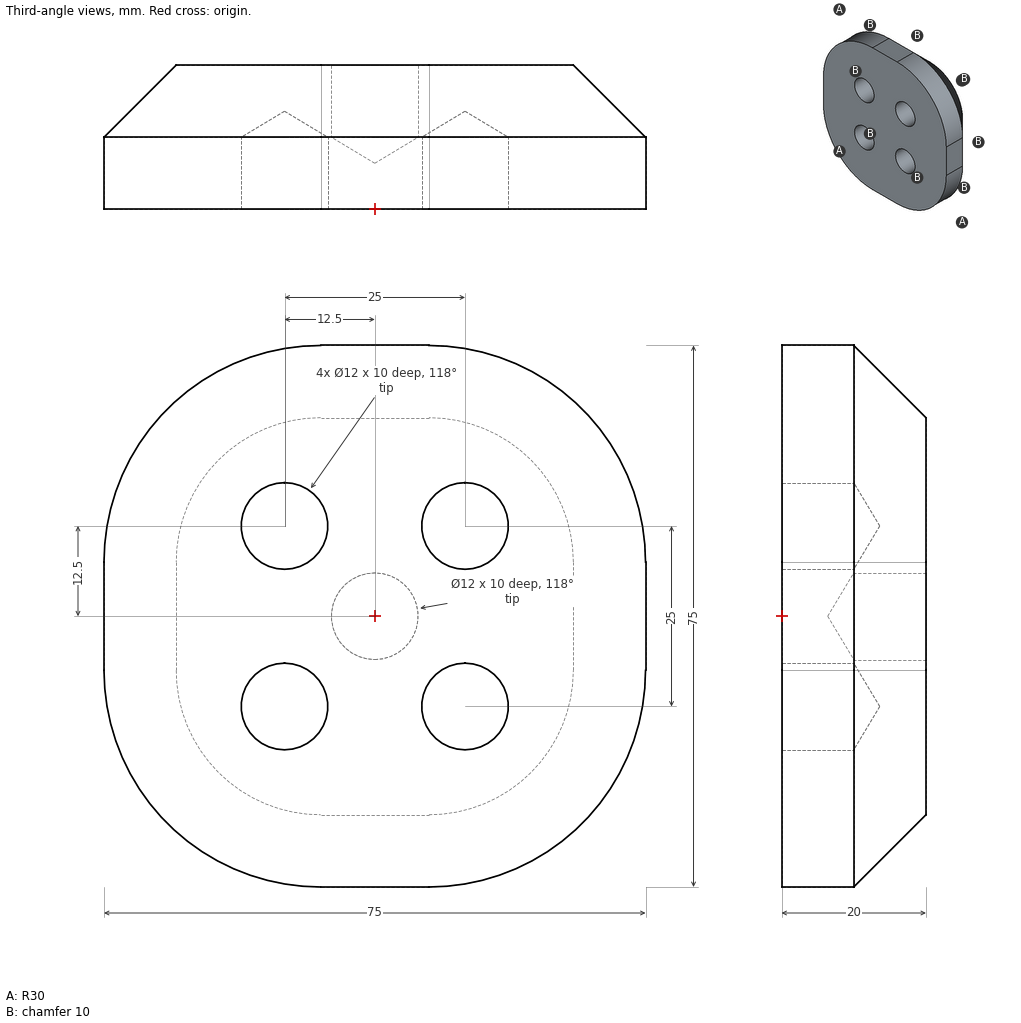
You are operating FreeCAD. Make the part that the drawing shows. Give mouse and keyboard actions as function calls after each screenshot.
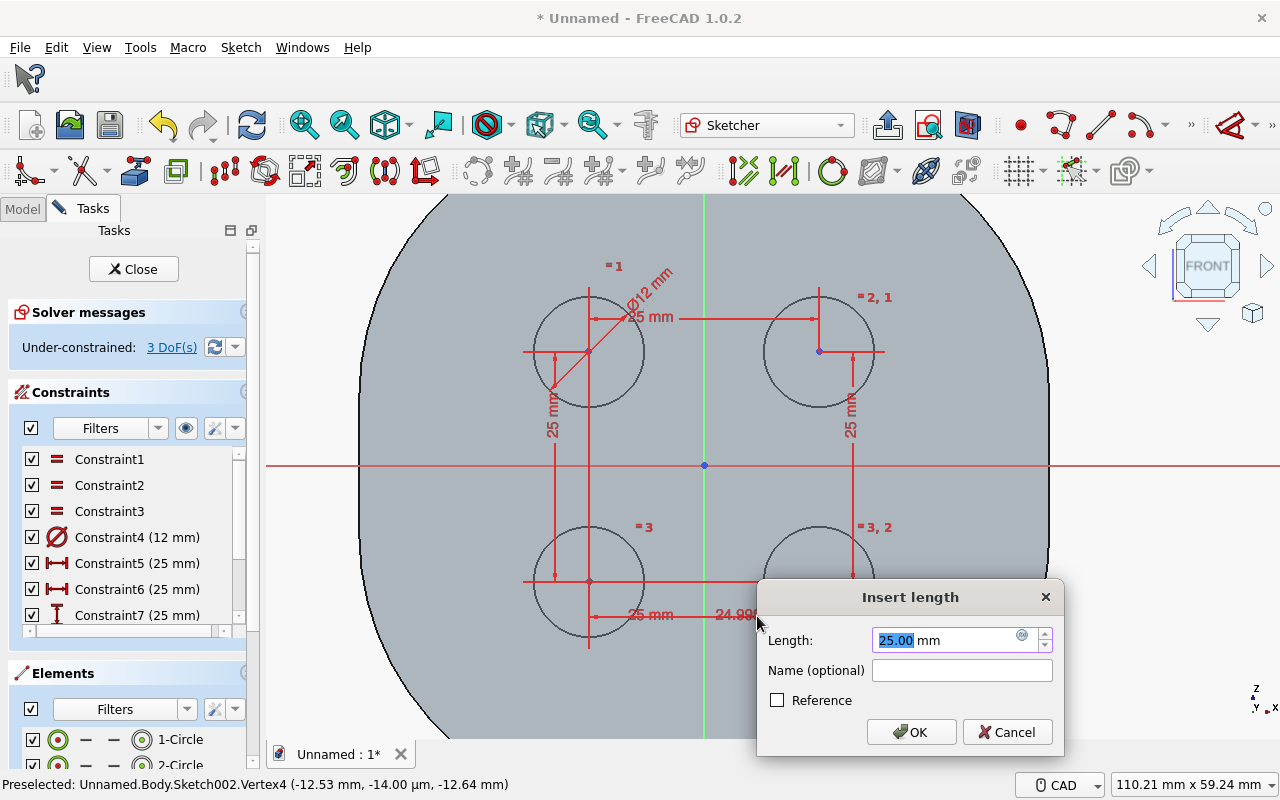
text(25)
key(Return)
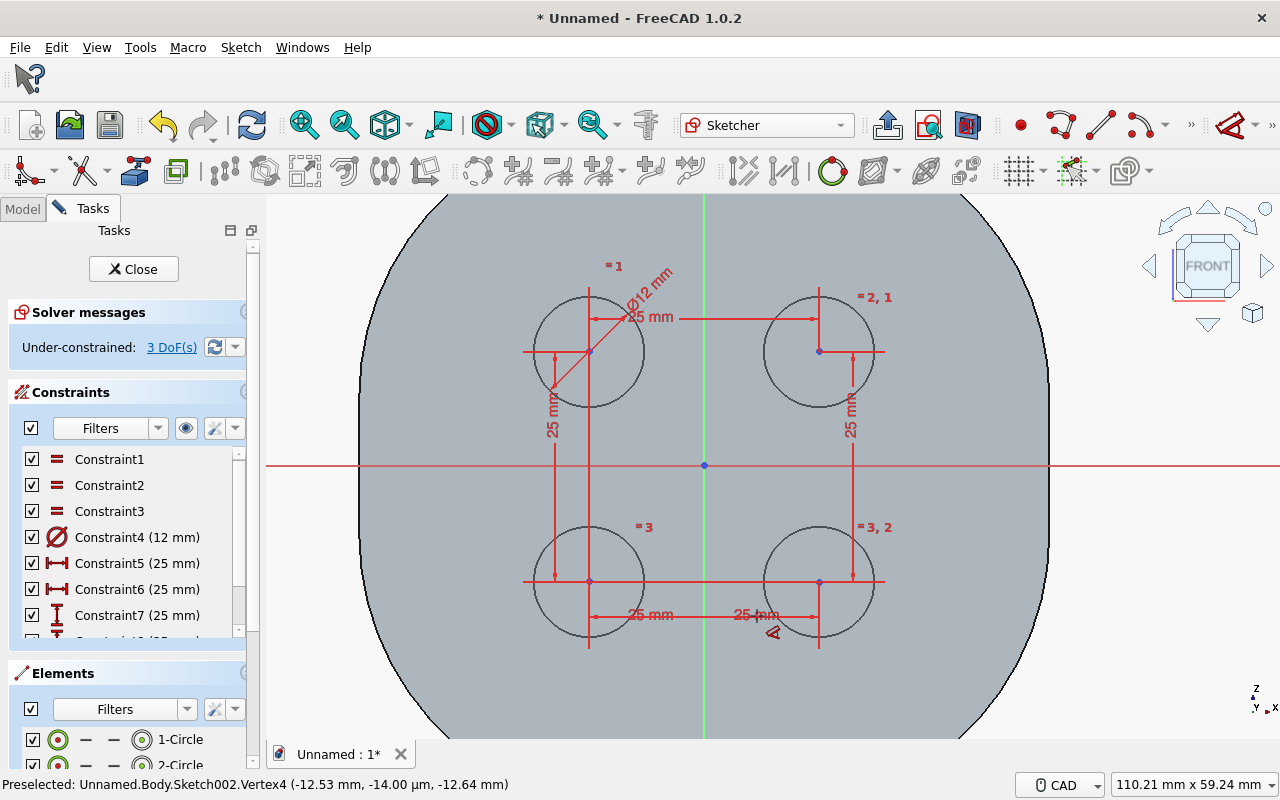
click(589, 352)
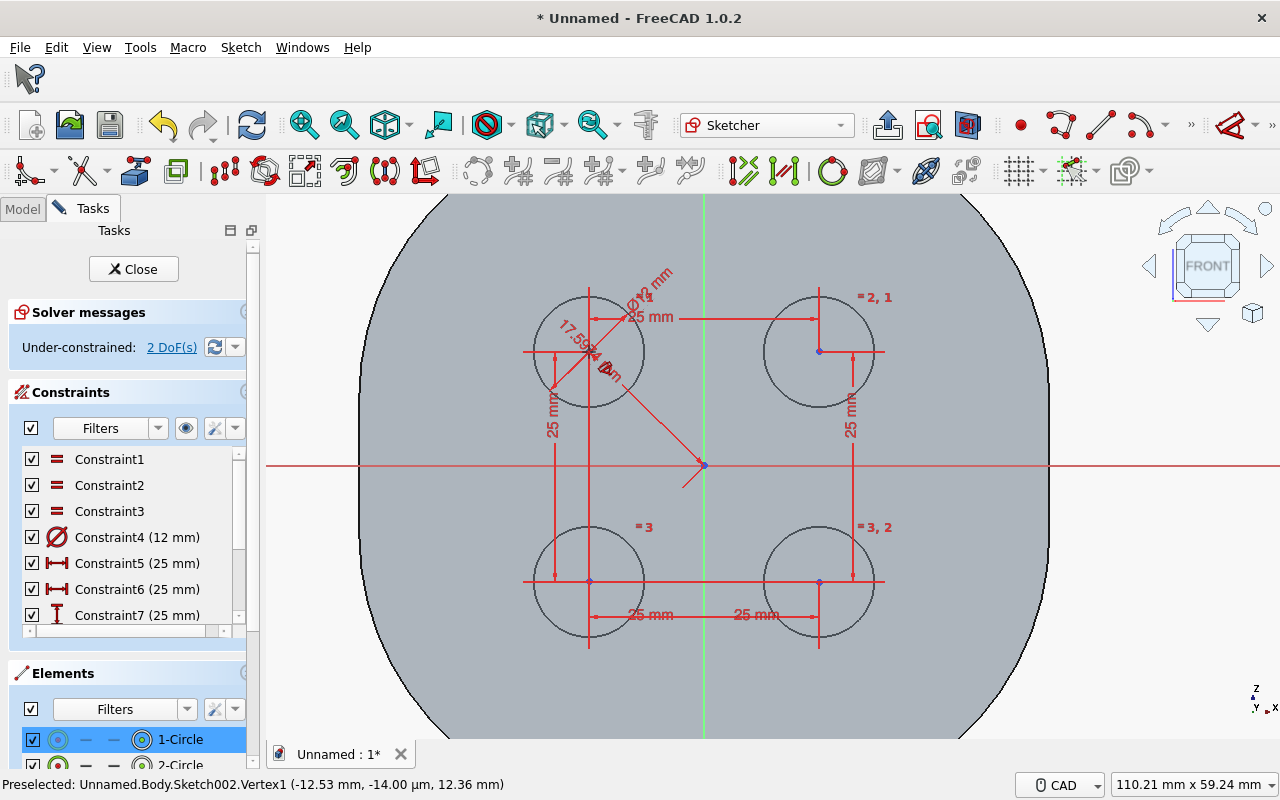
click(589, 582)
click(555, 520)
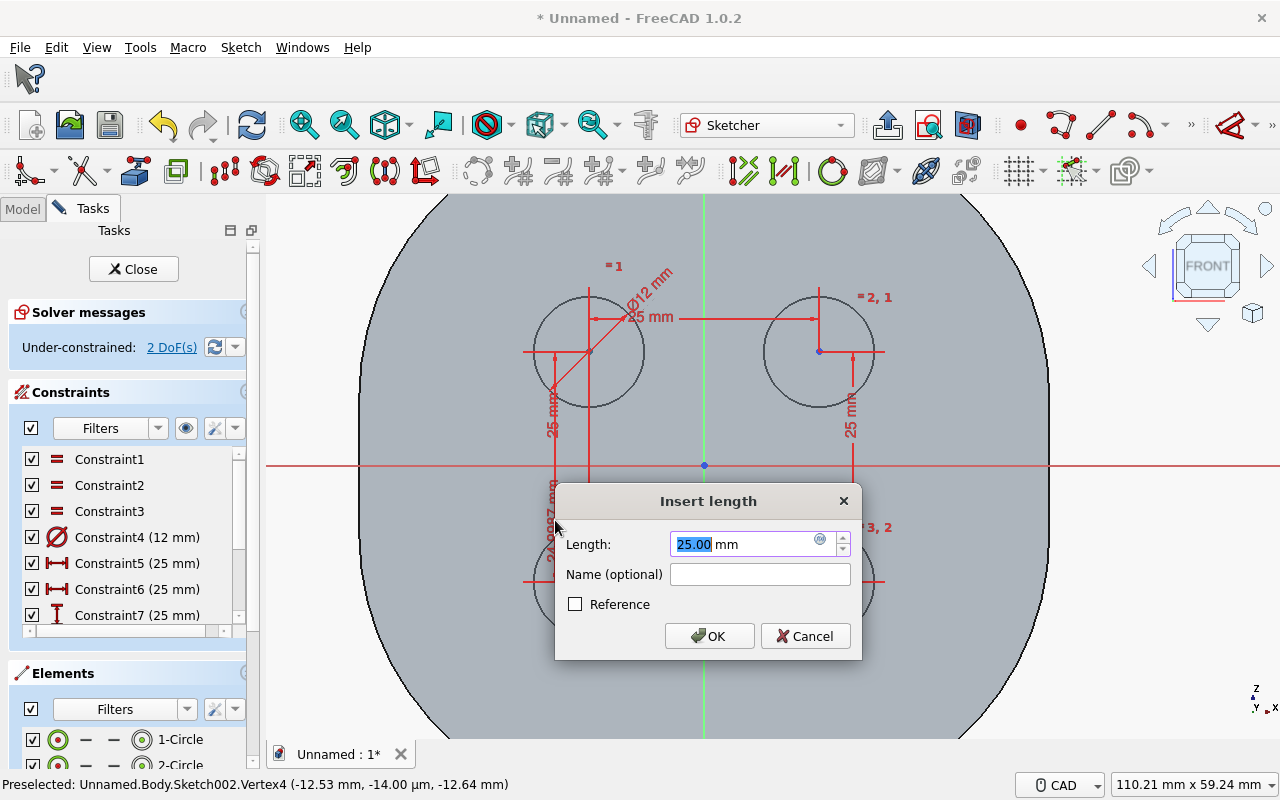
text(25)
key(Return)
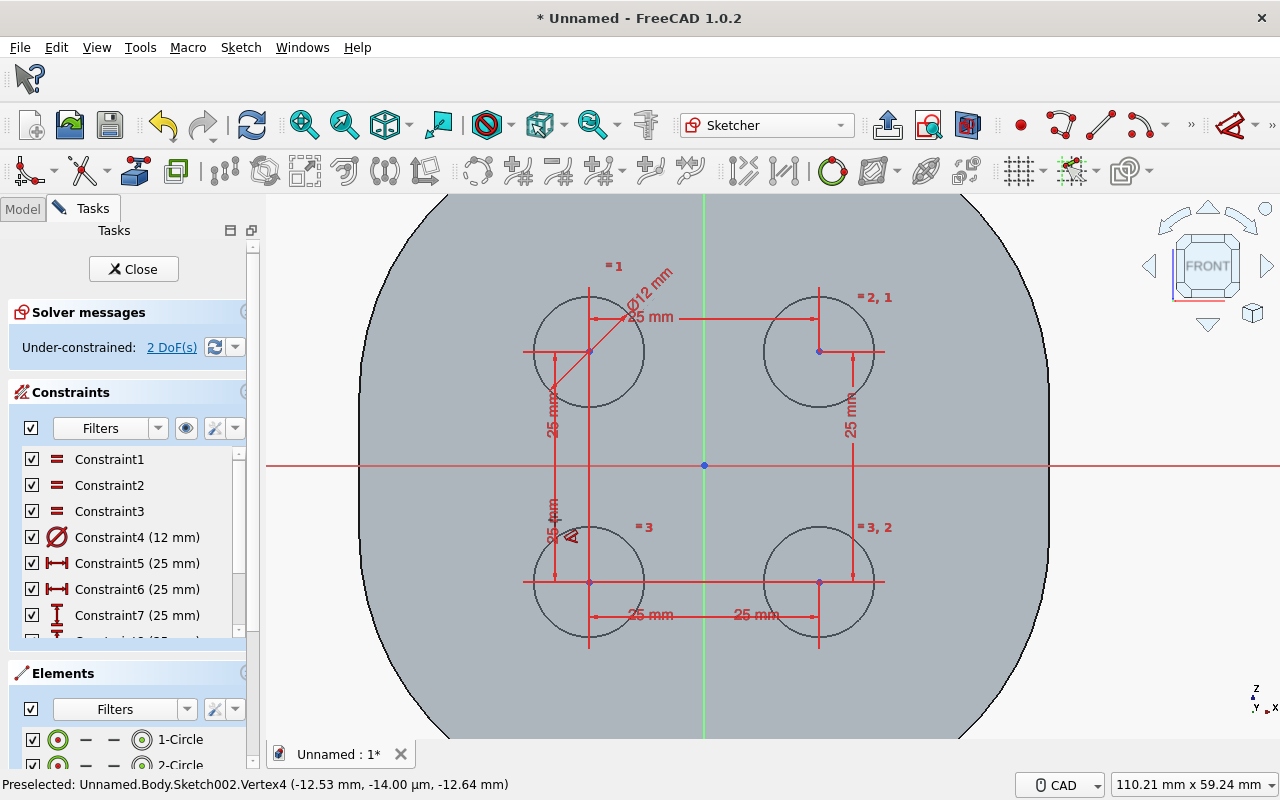
click(589, 352)
click(647, 500)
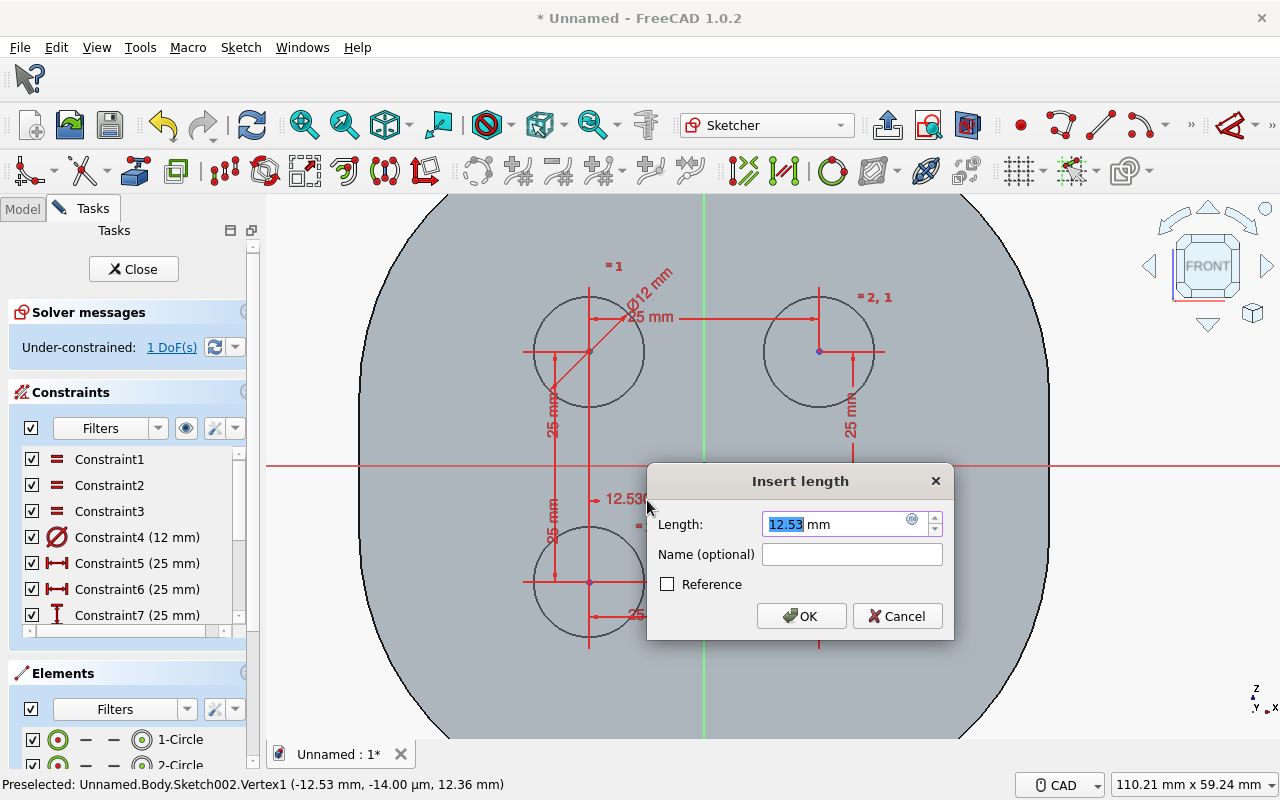
text(12.5)
key(Return)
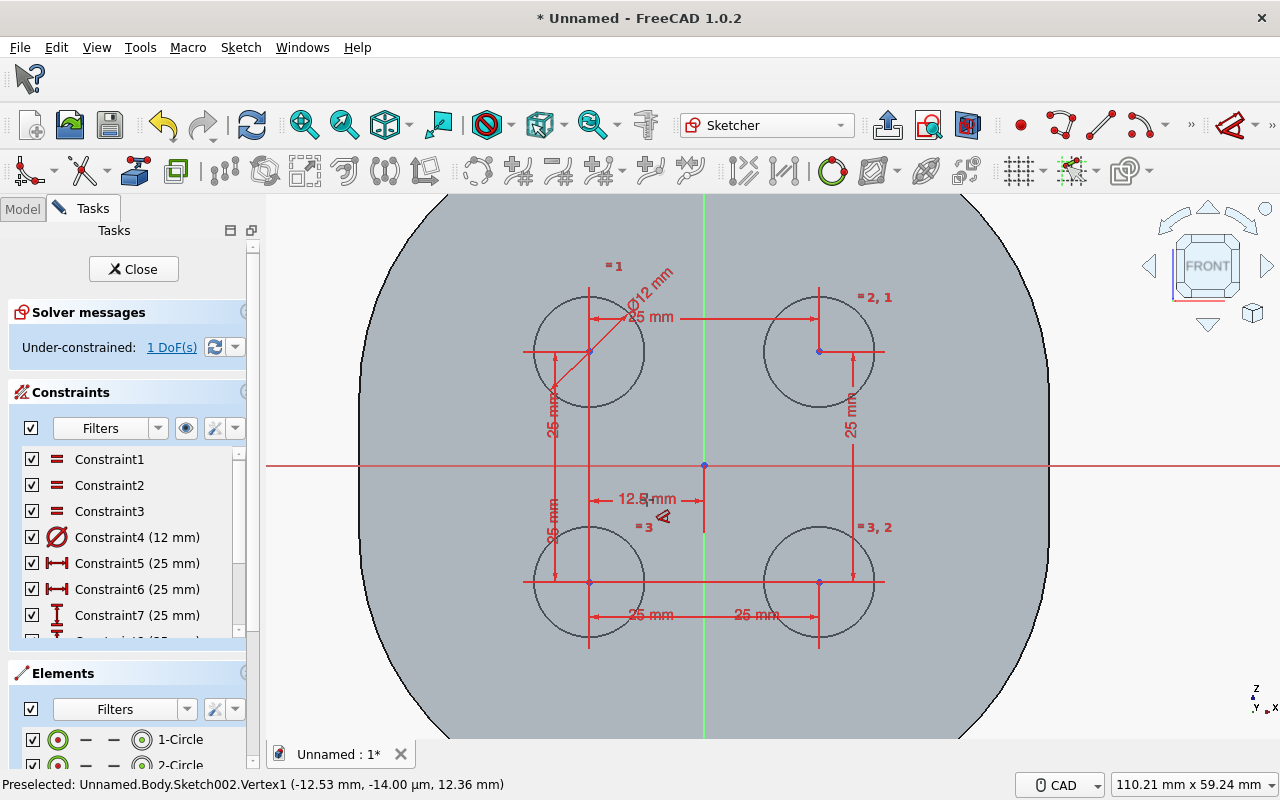
click(589, 352)
click(555, 435)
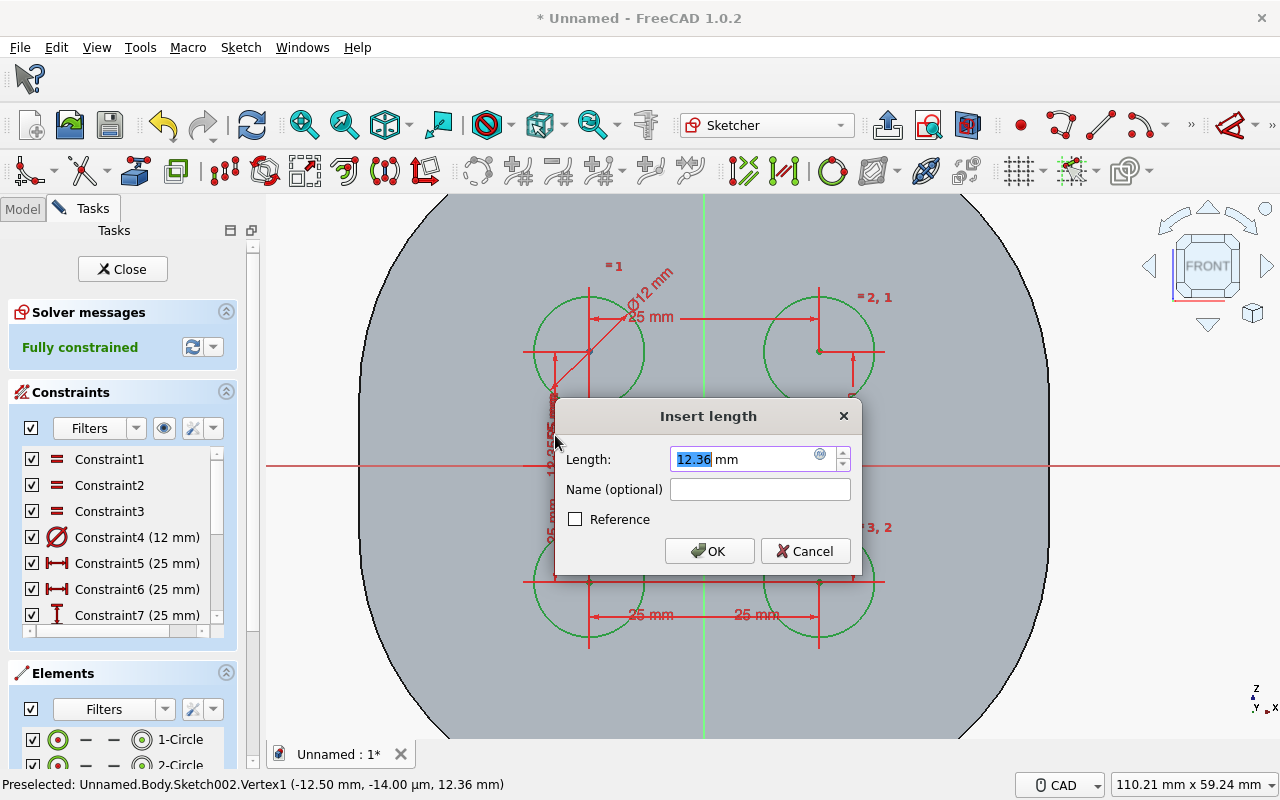
text(12.5)
key(Return)
key(Escape)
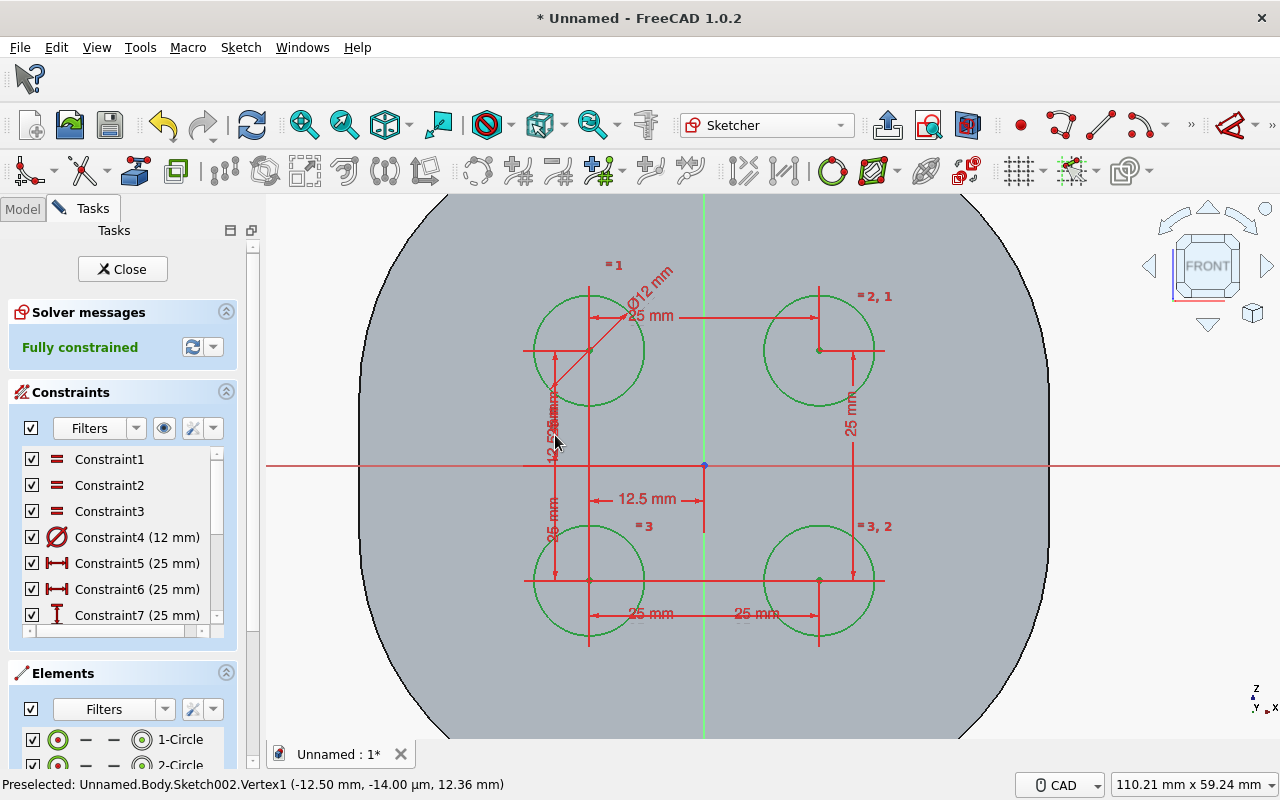
click(123, 269)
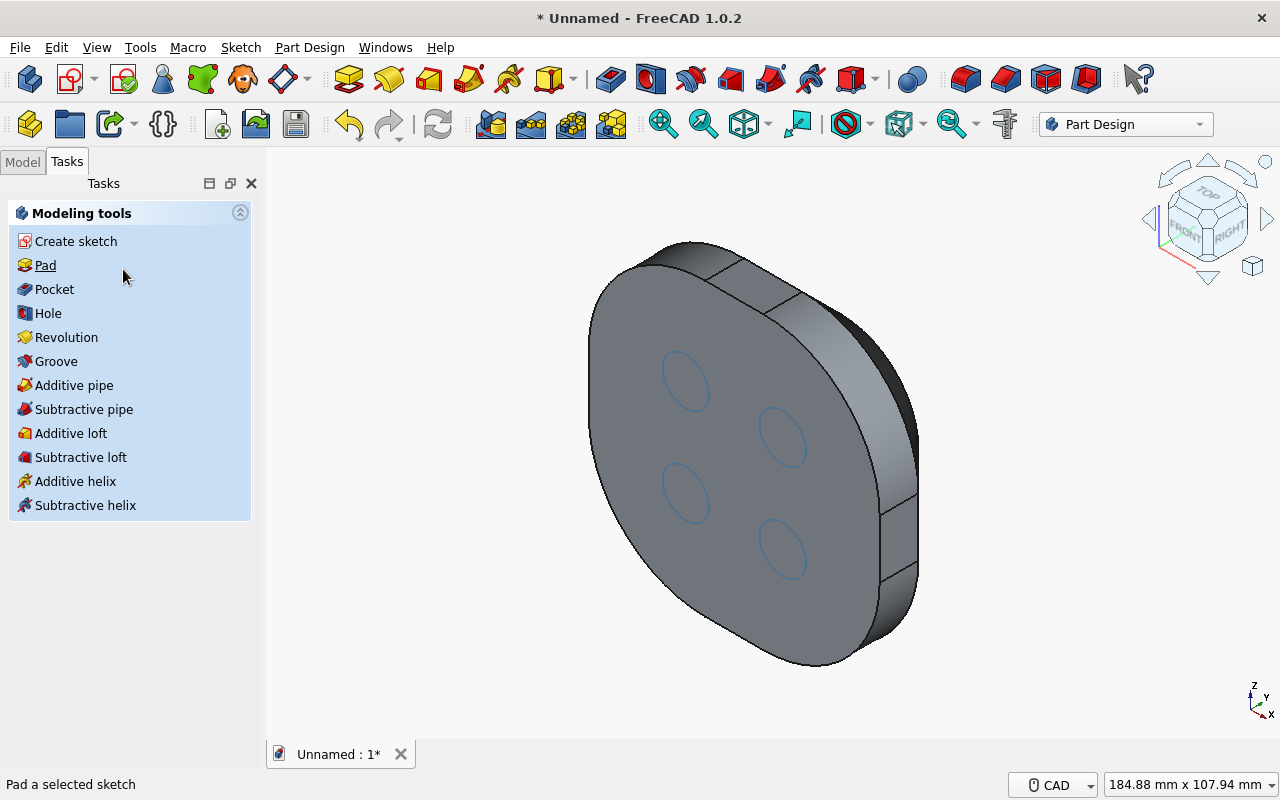
click(652, 80)